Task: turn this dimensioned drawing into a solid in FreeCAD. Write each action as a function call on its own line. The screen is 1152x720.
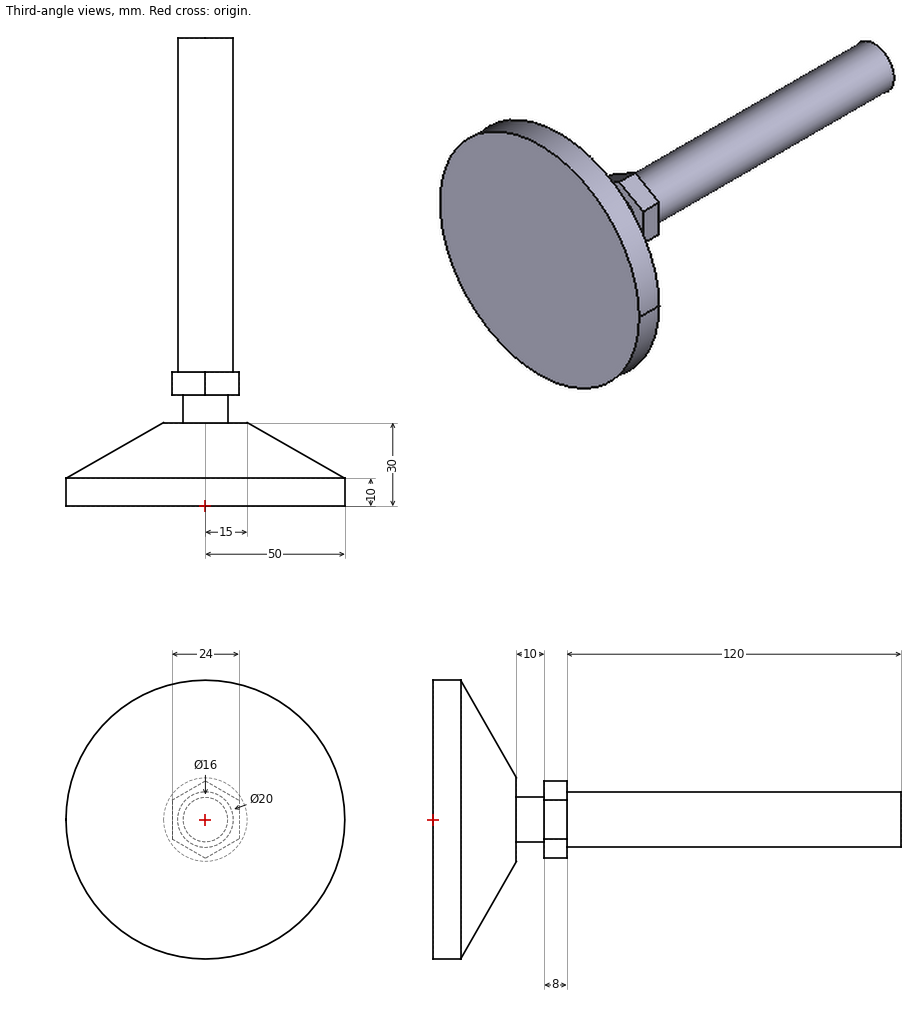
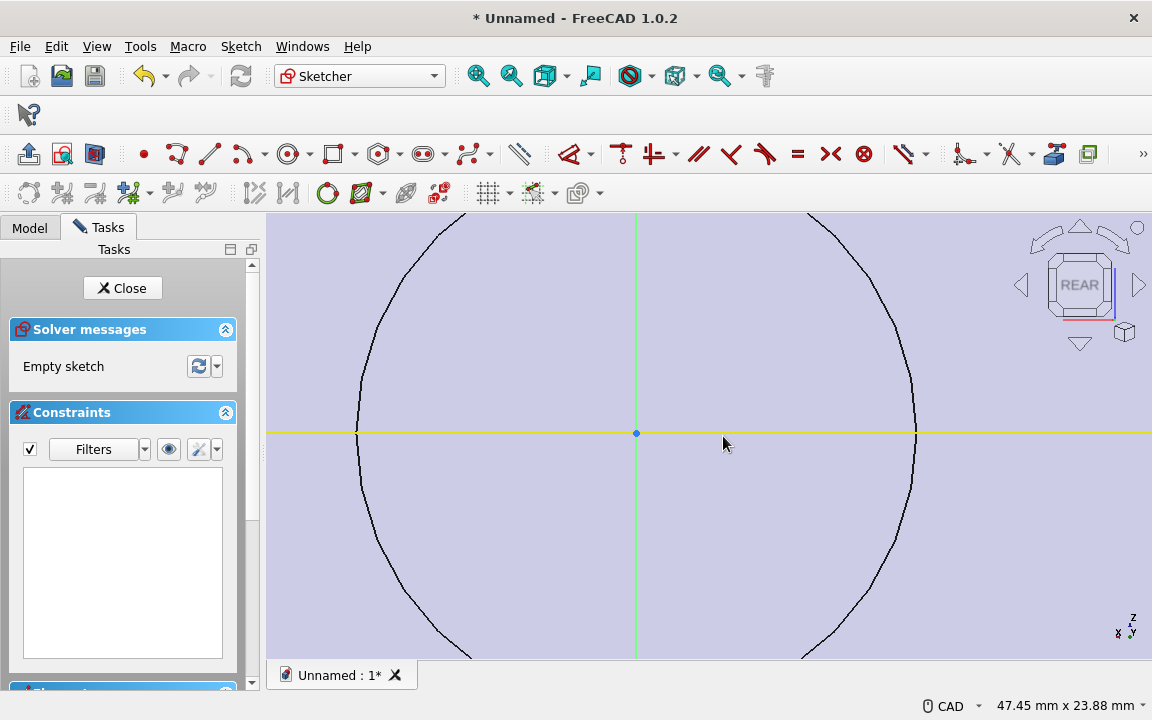
key(g)
key(c)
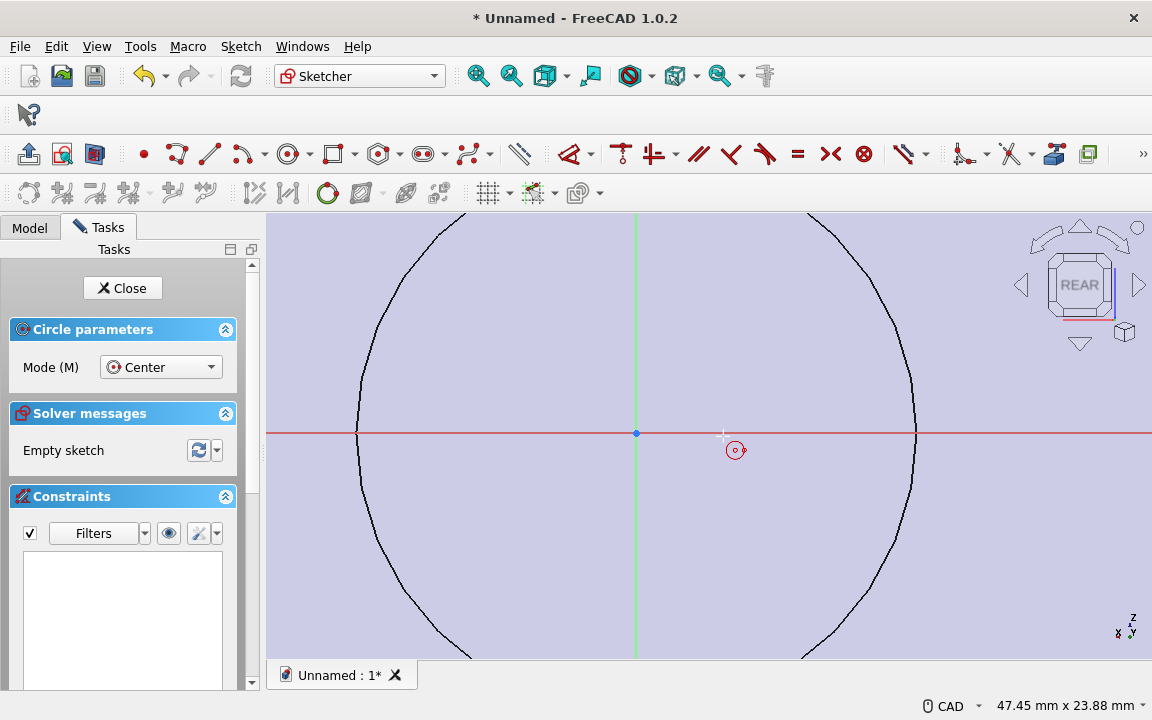
click(636, 433)
move(742, 328)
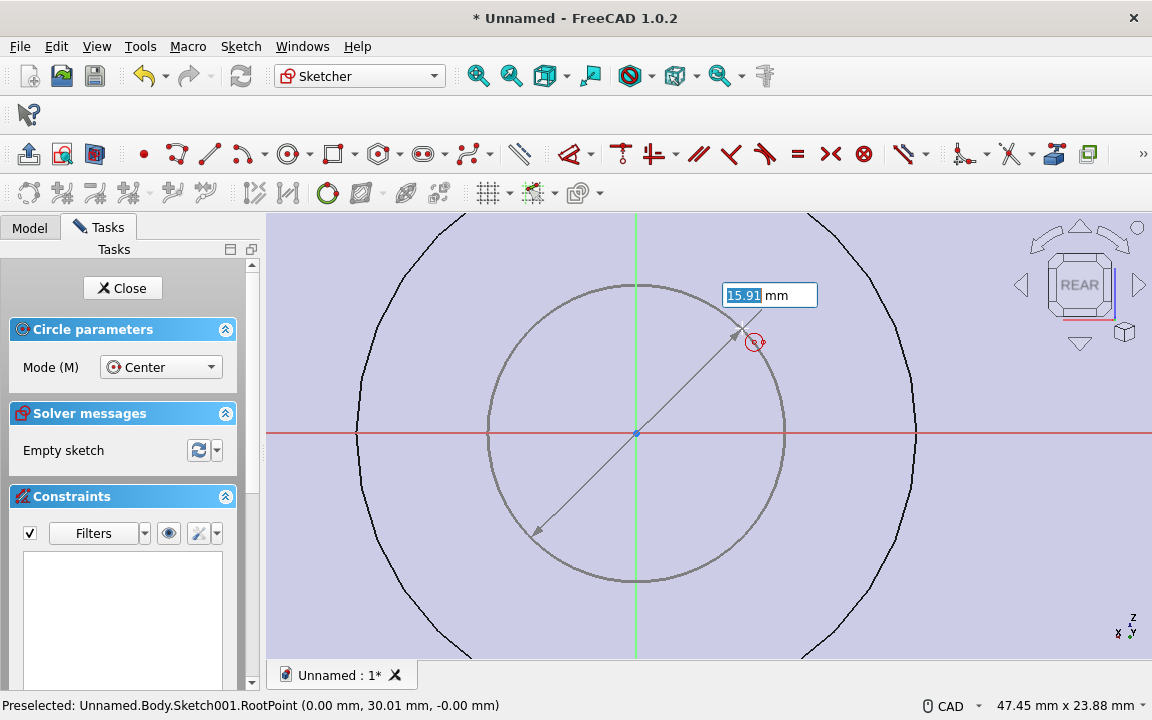
text(16)
key(Return)
key(Escape)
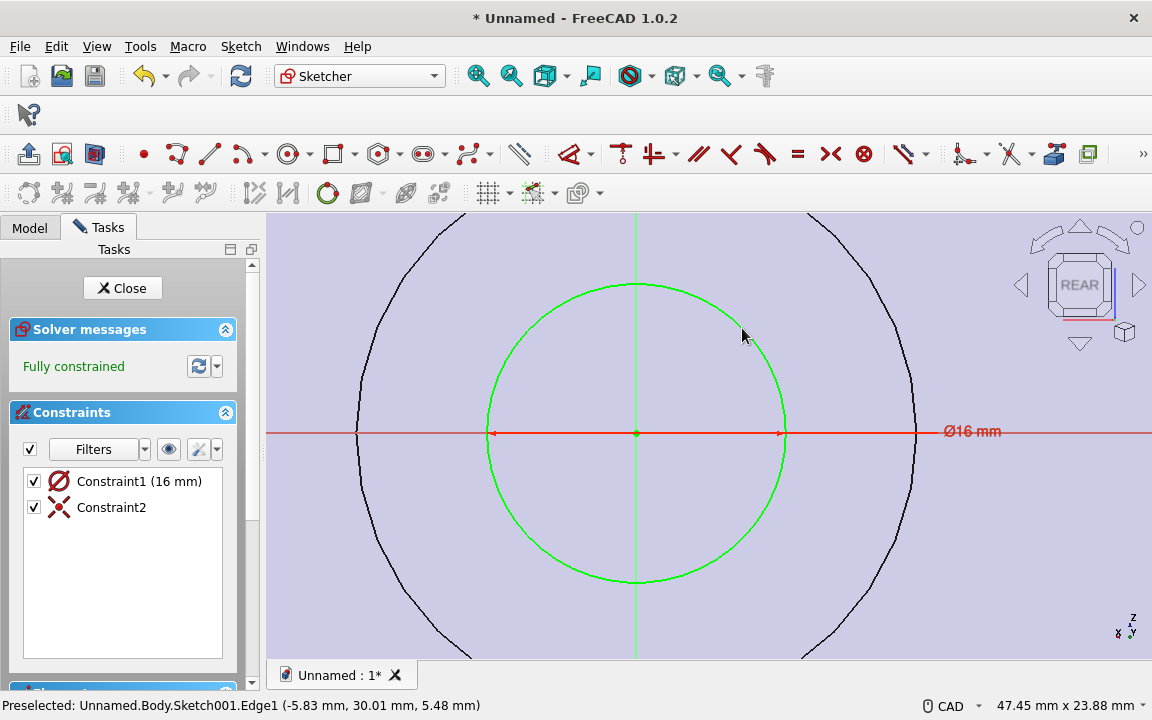
click(123, 288)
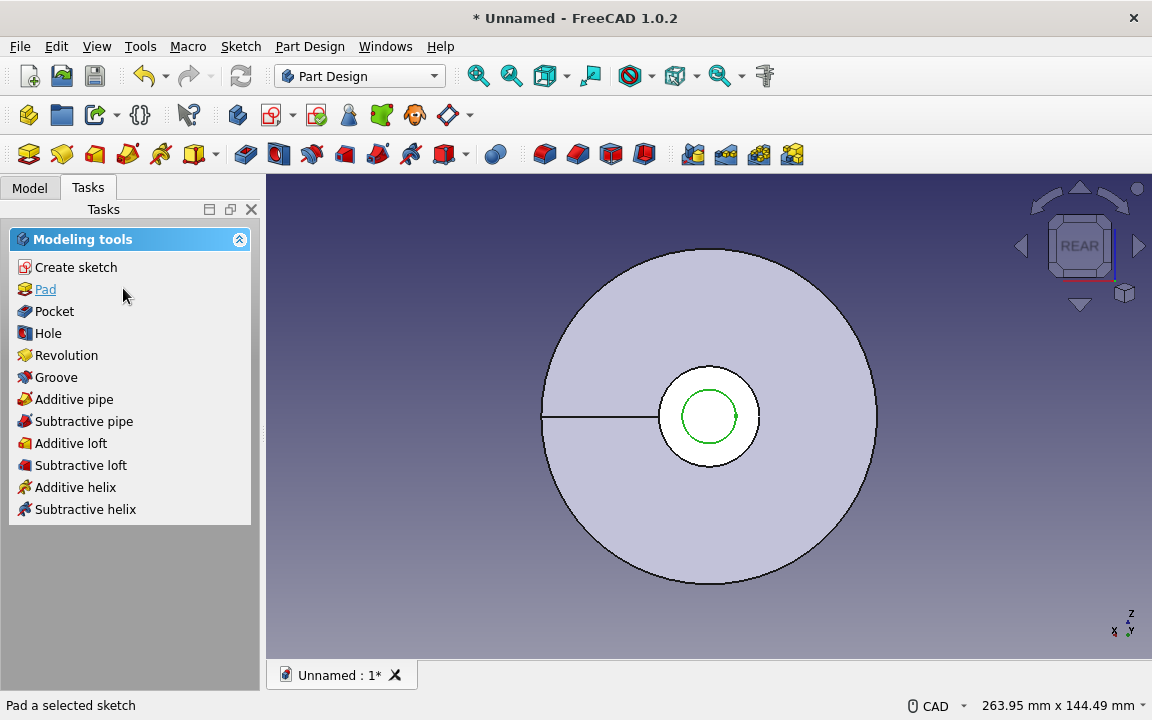
click(29, 154)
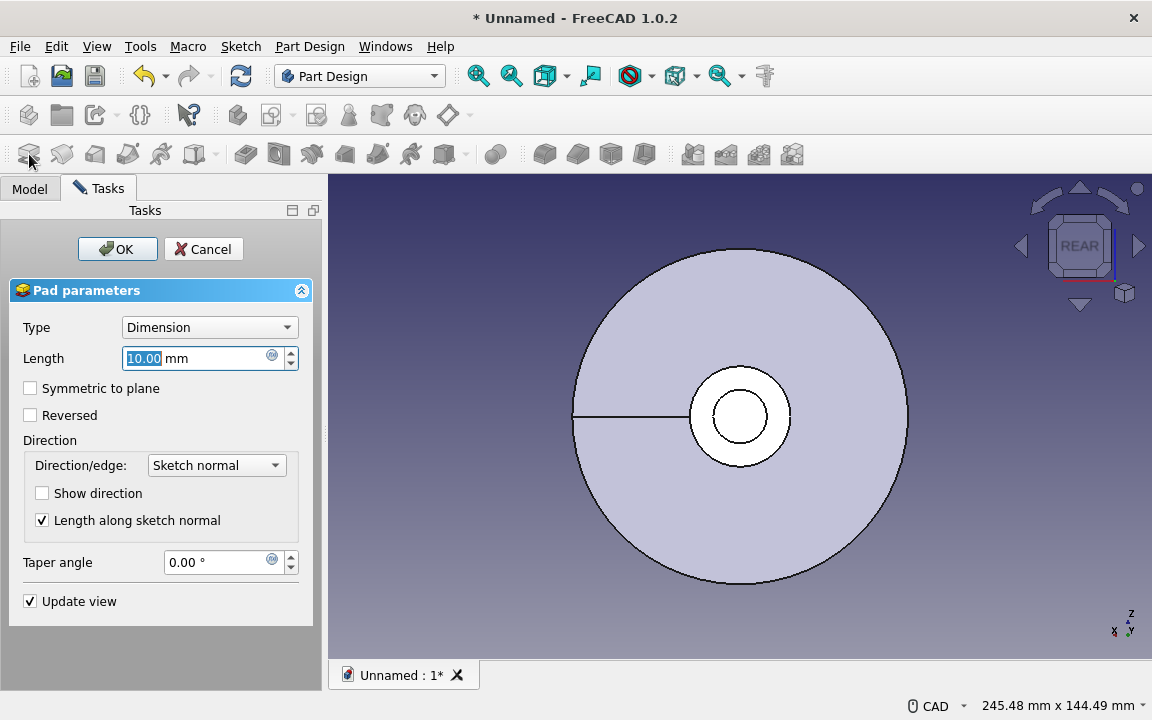
text(10)
key(Tab)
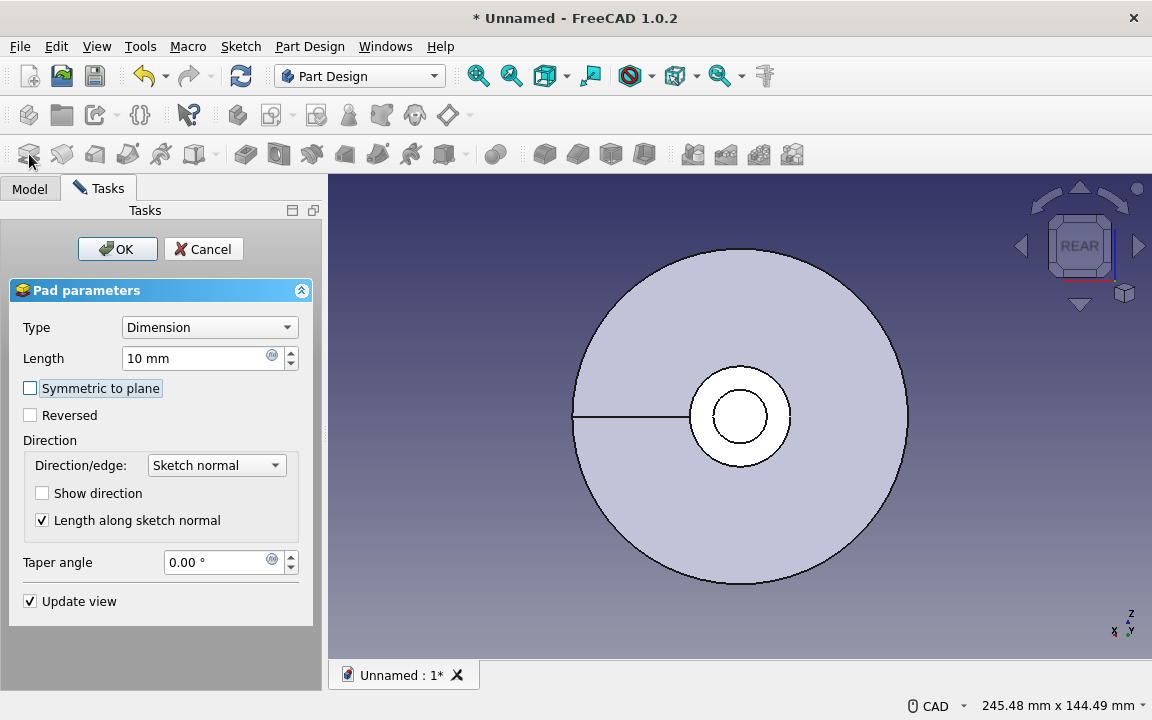
click(118, 249)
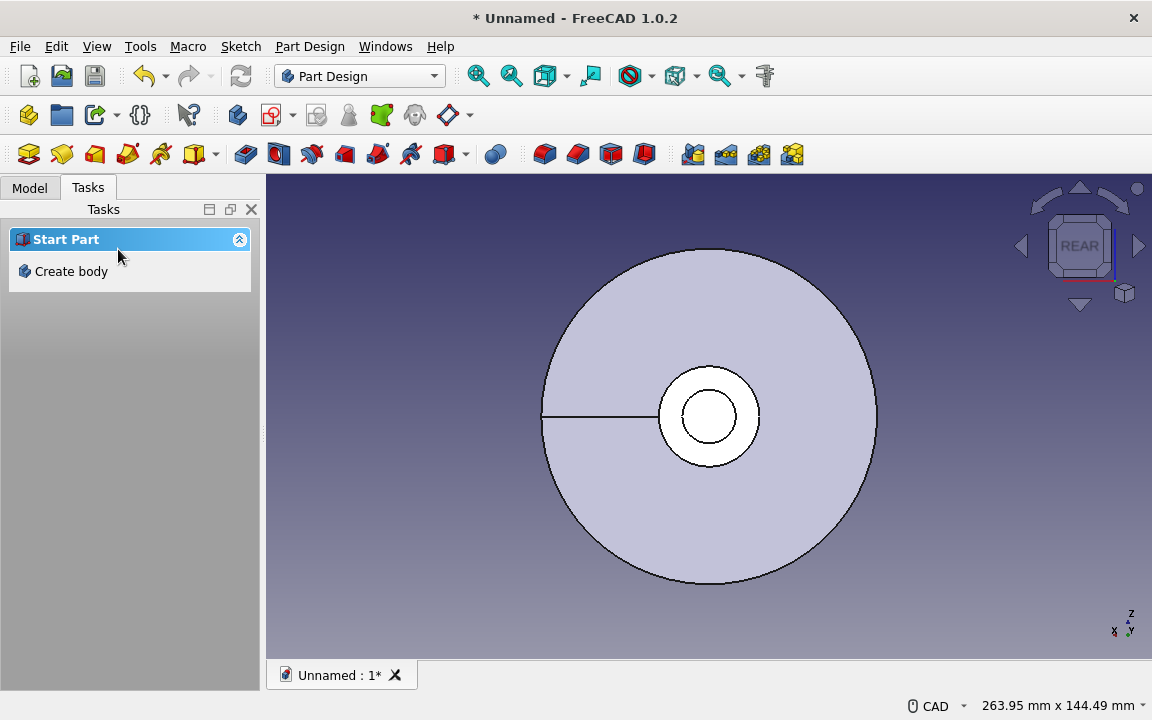
click(709, 415)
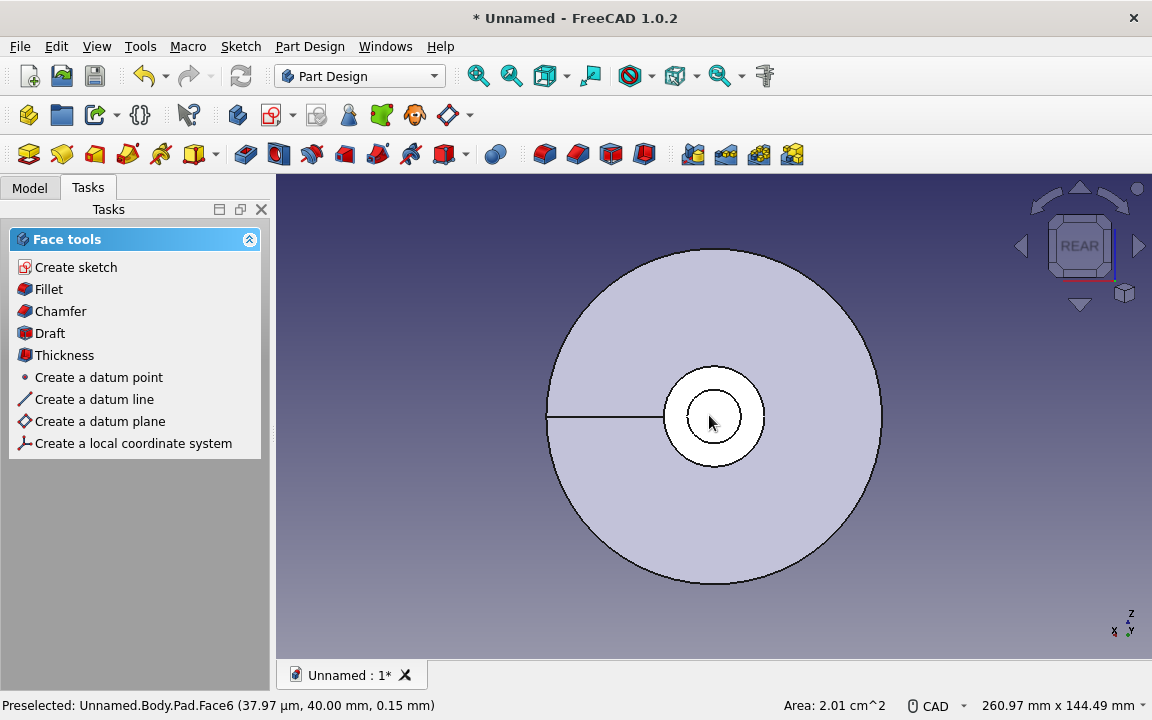
click(270, 116)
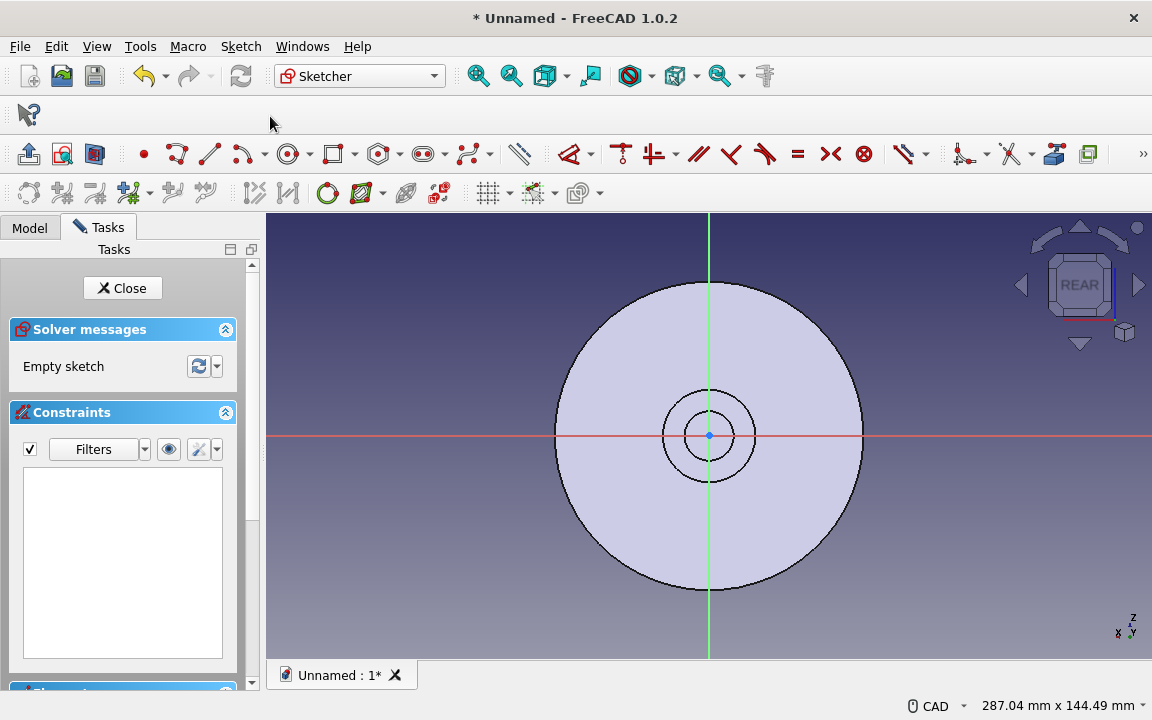
scroll(739, 436, up, 6)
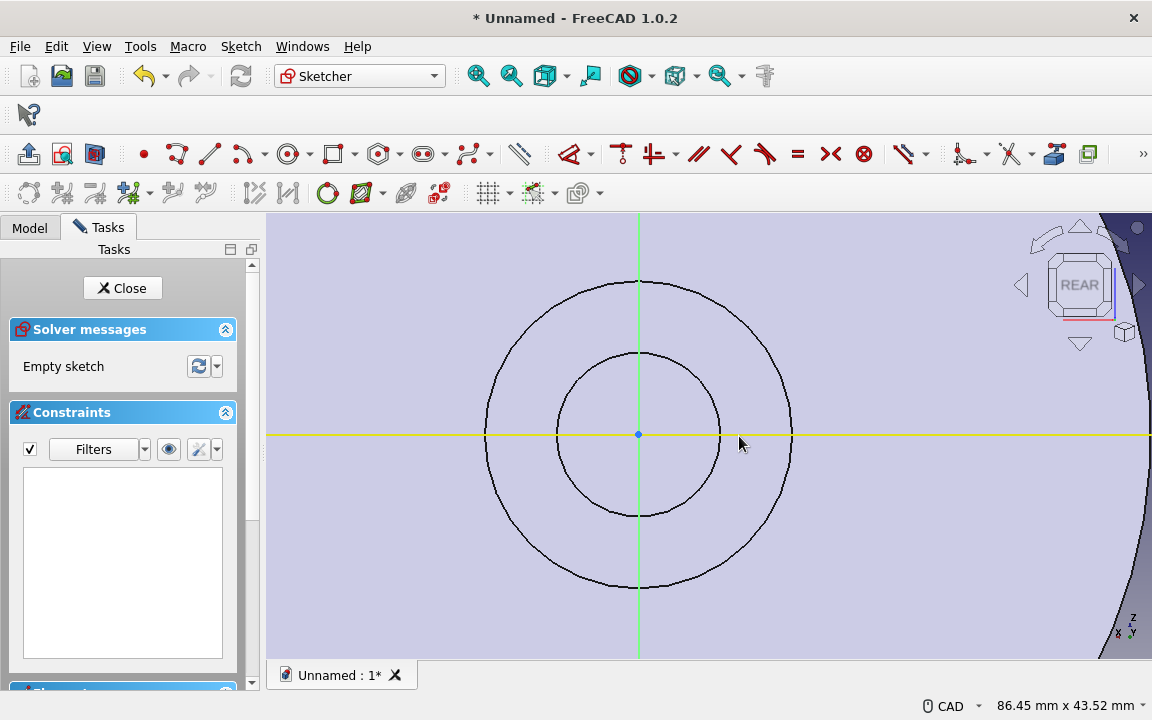
key(g)
key(p)
key(6)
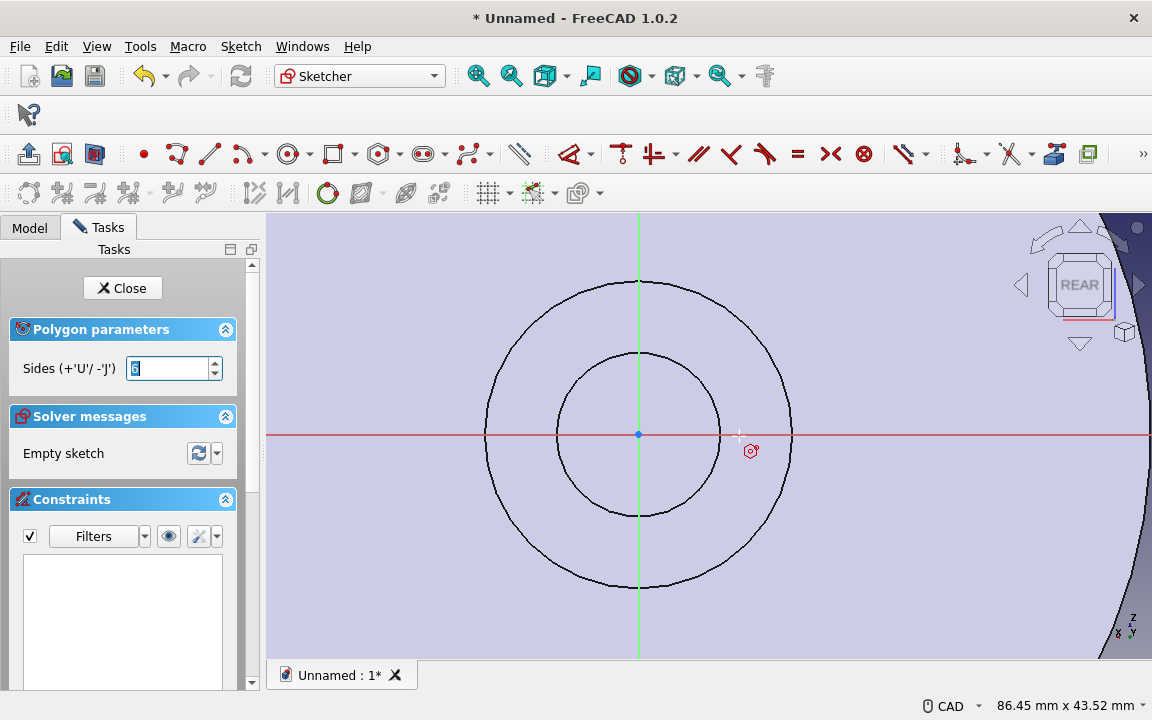
click(639, 435)